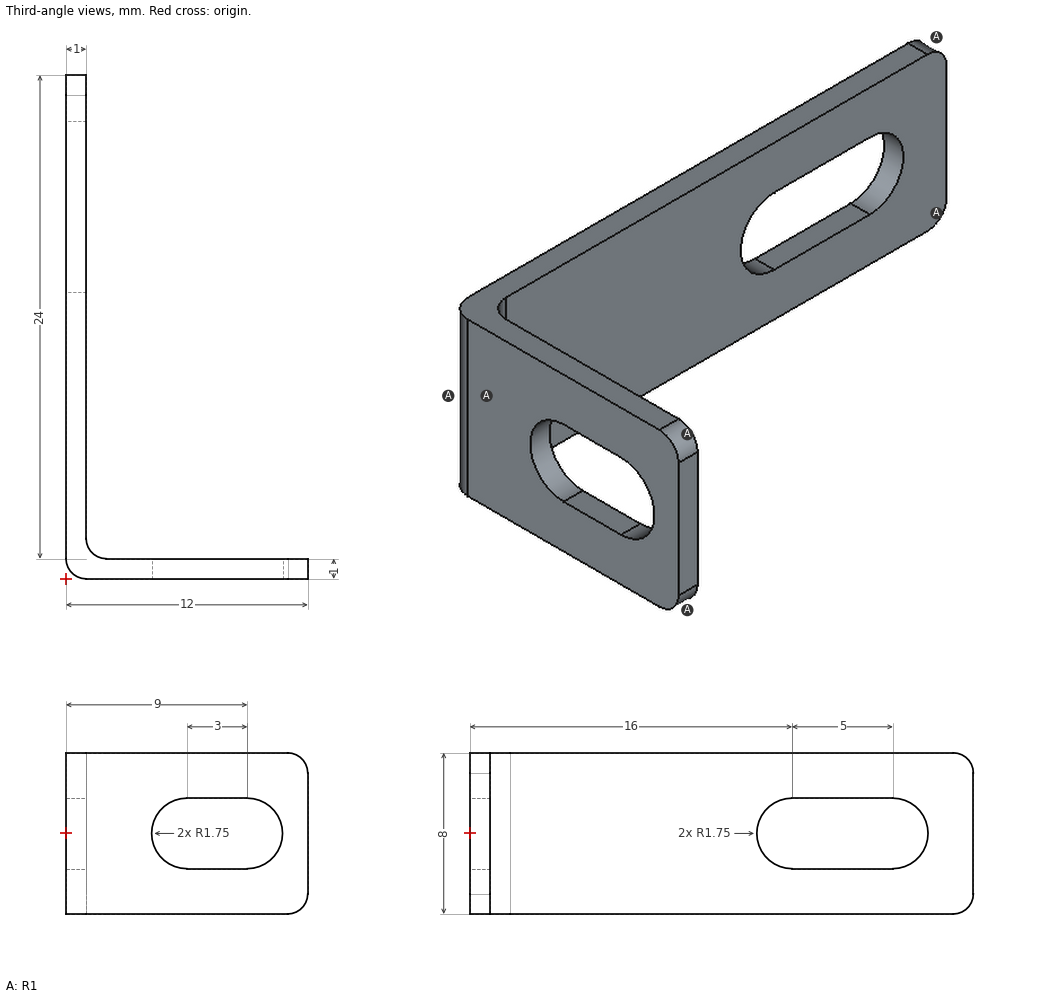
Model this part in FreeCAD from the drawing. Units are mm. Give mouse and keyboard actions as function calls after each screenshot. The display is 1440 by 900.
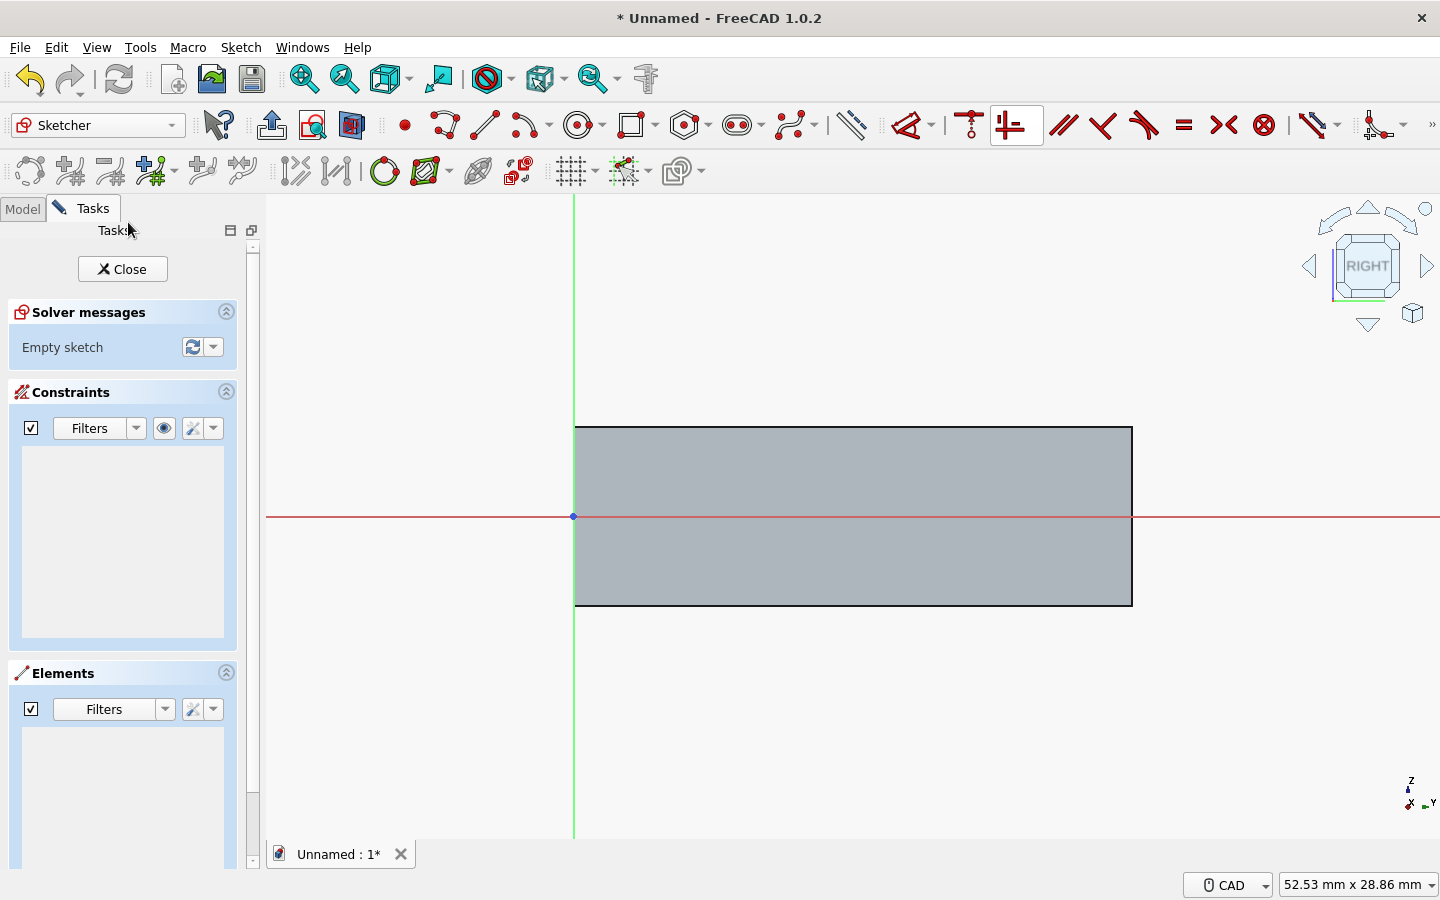
scroll(1074, 516, up, 6)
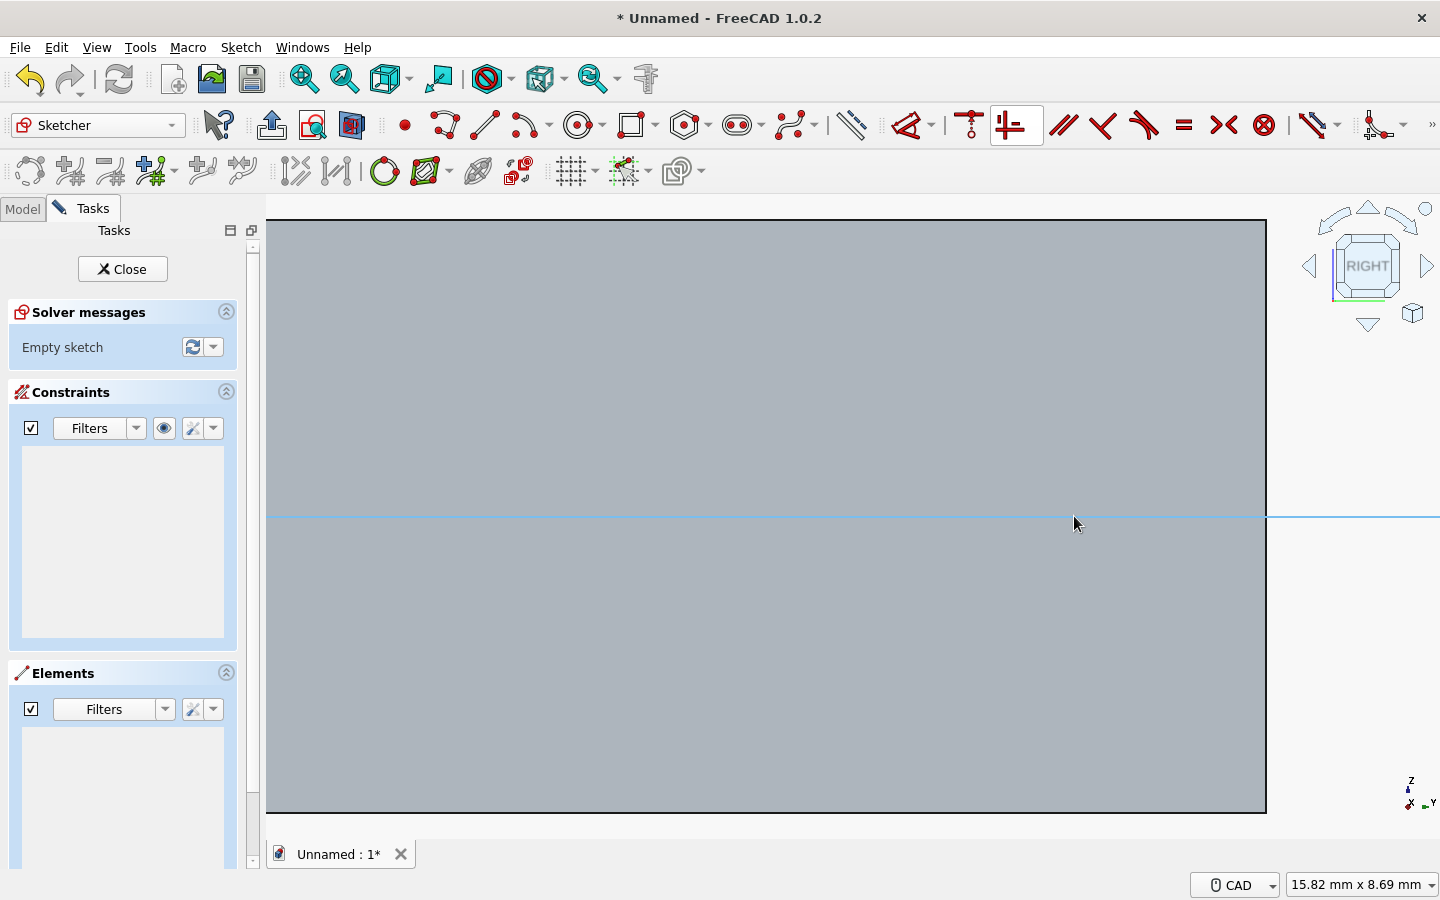
key(g)
key(s)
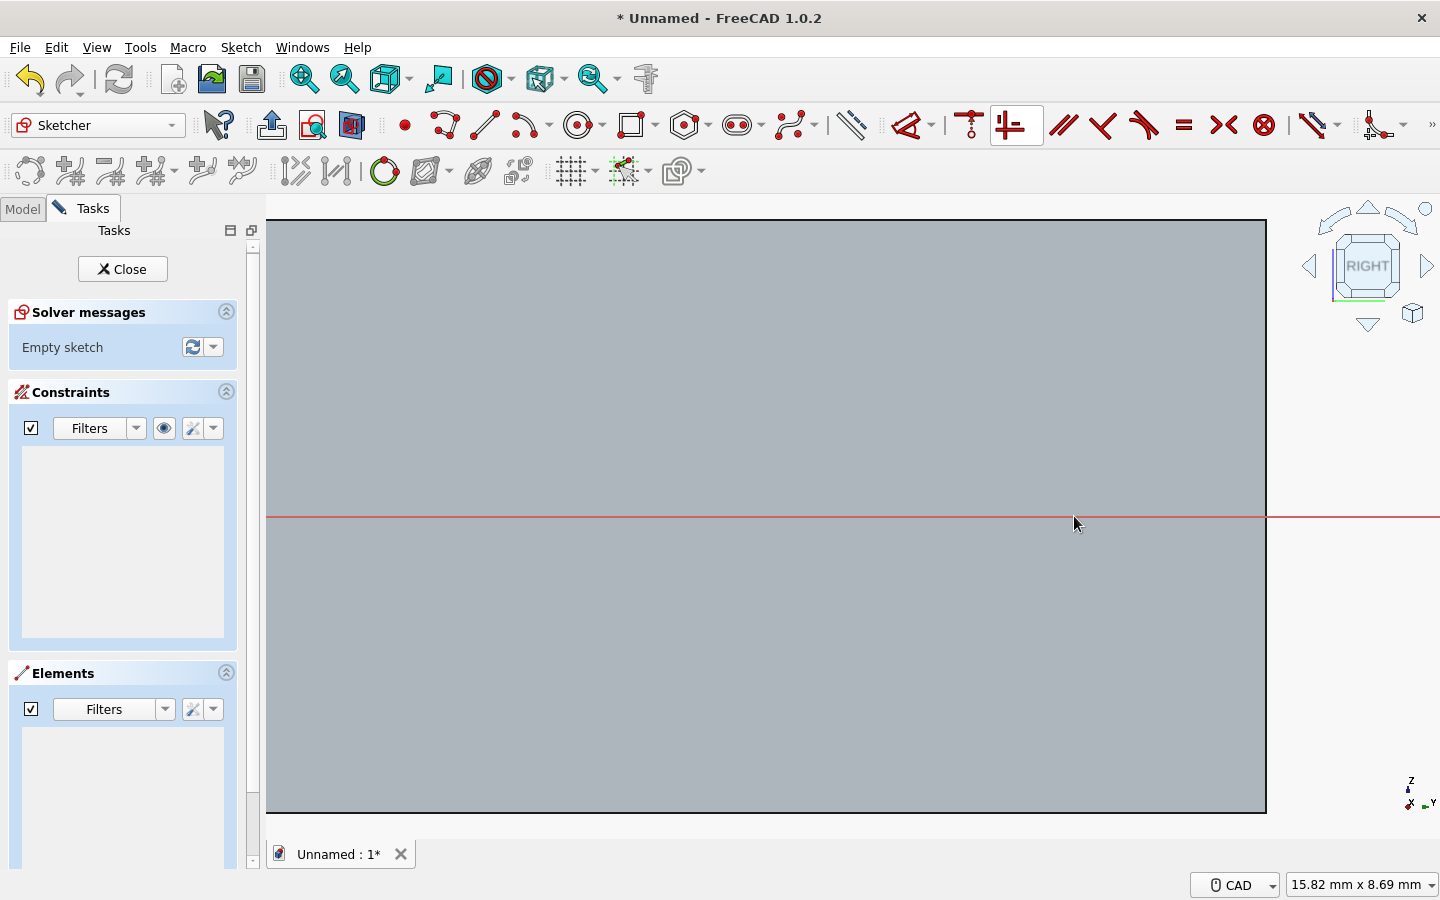
click(598, 516)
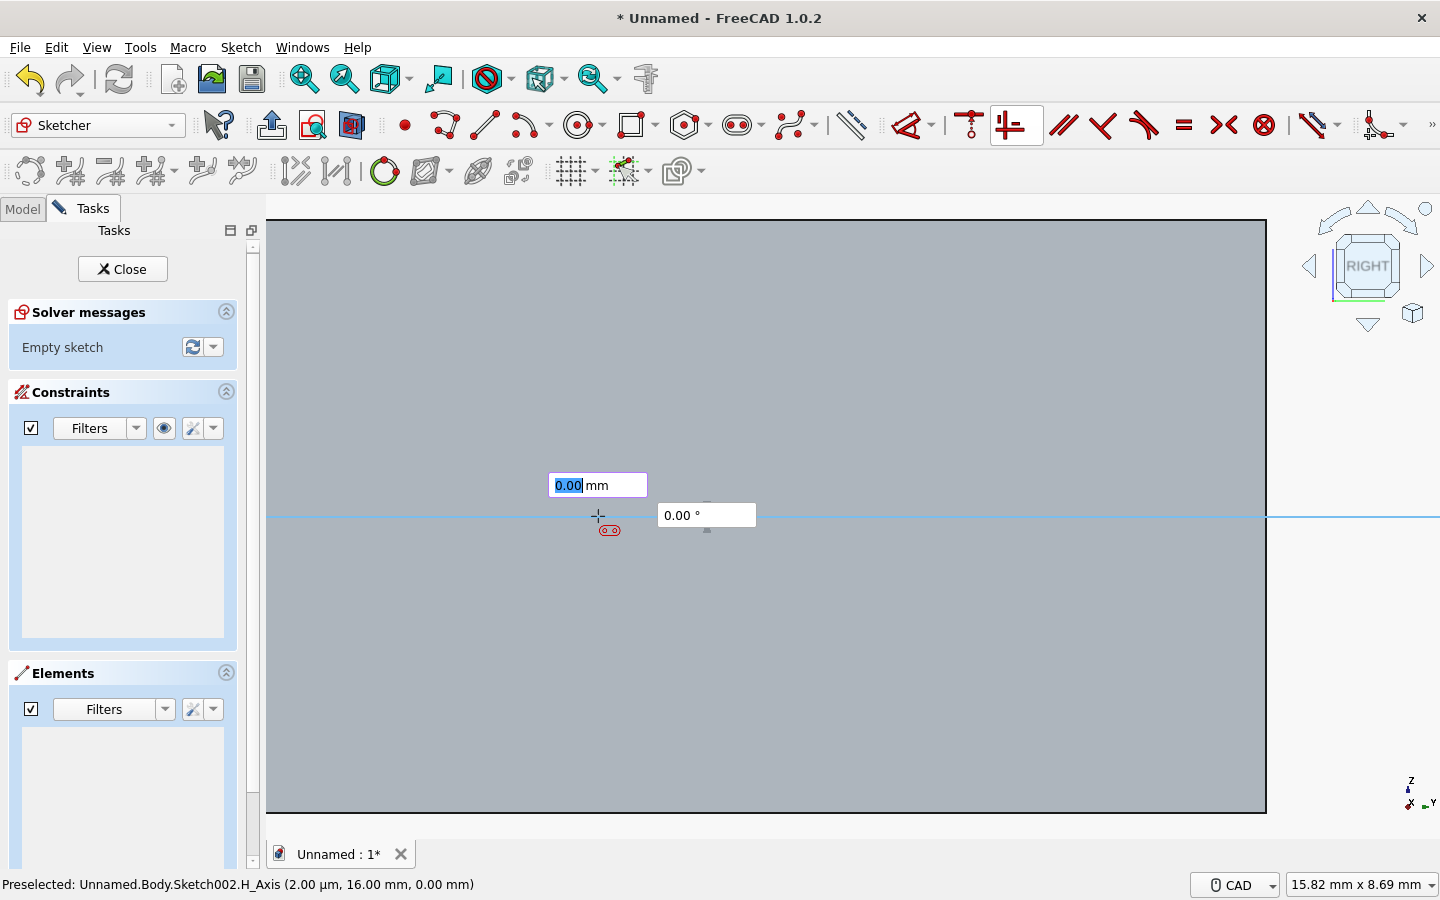
click(969, 508)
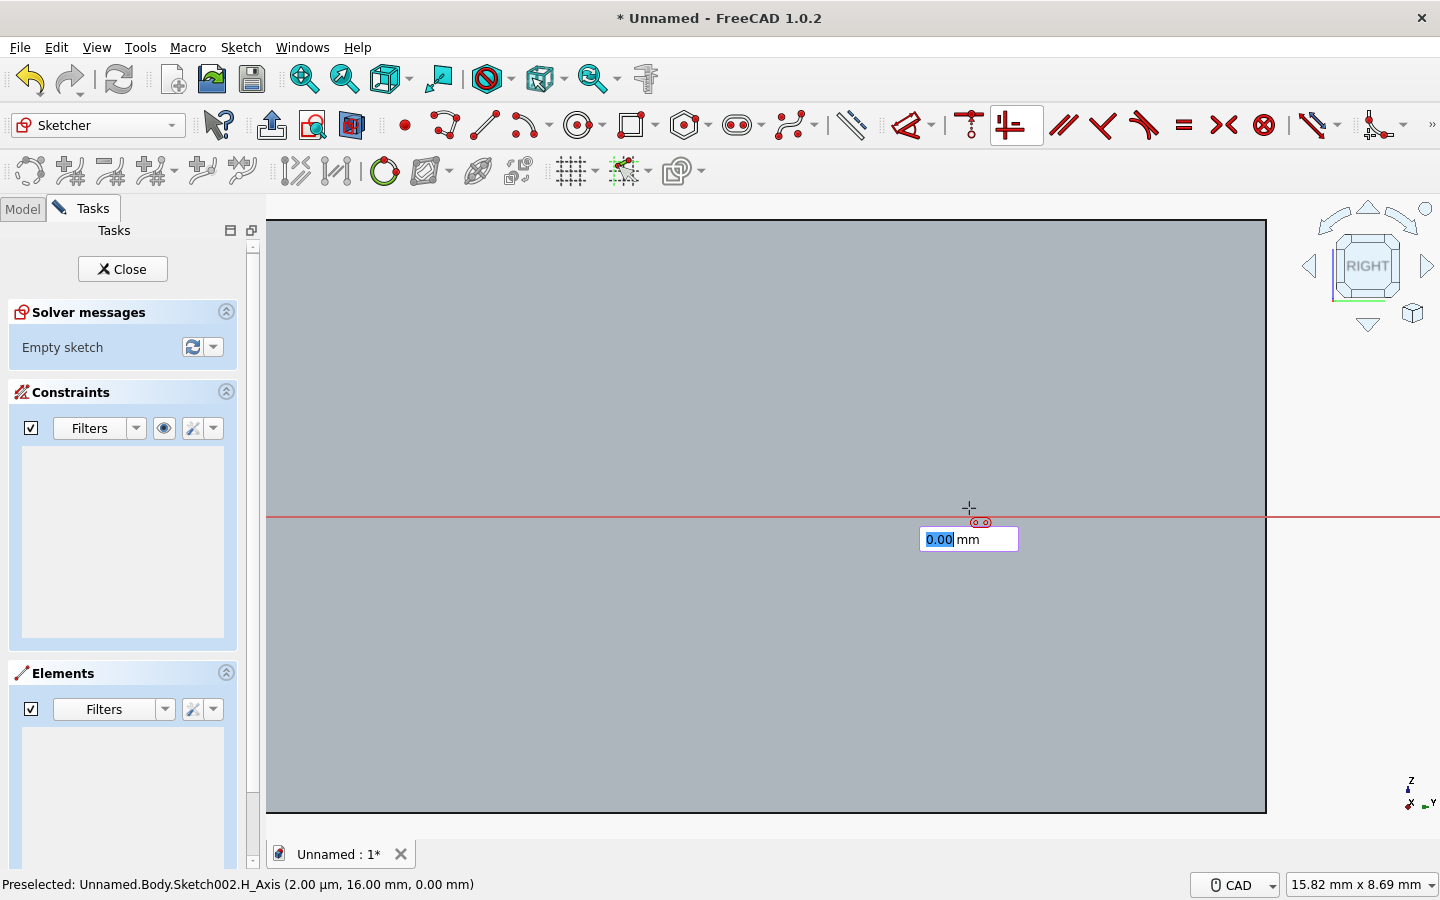
click(784, 646)
key(Escape)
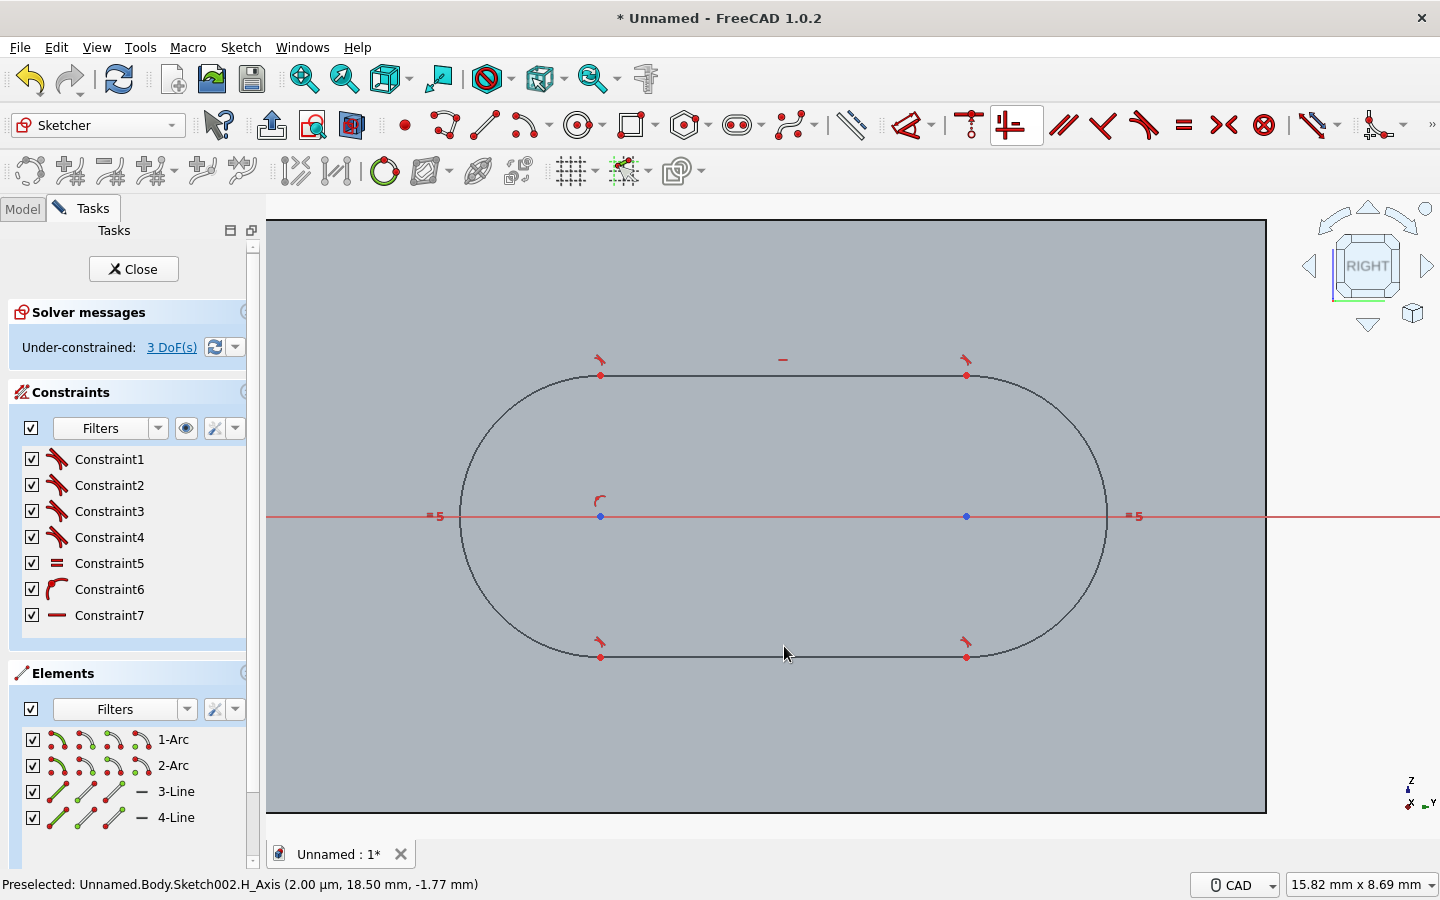
key(d)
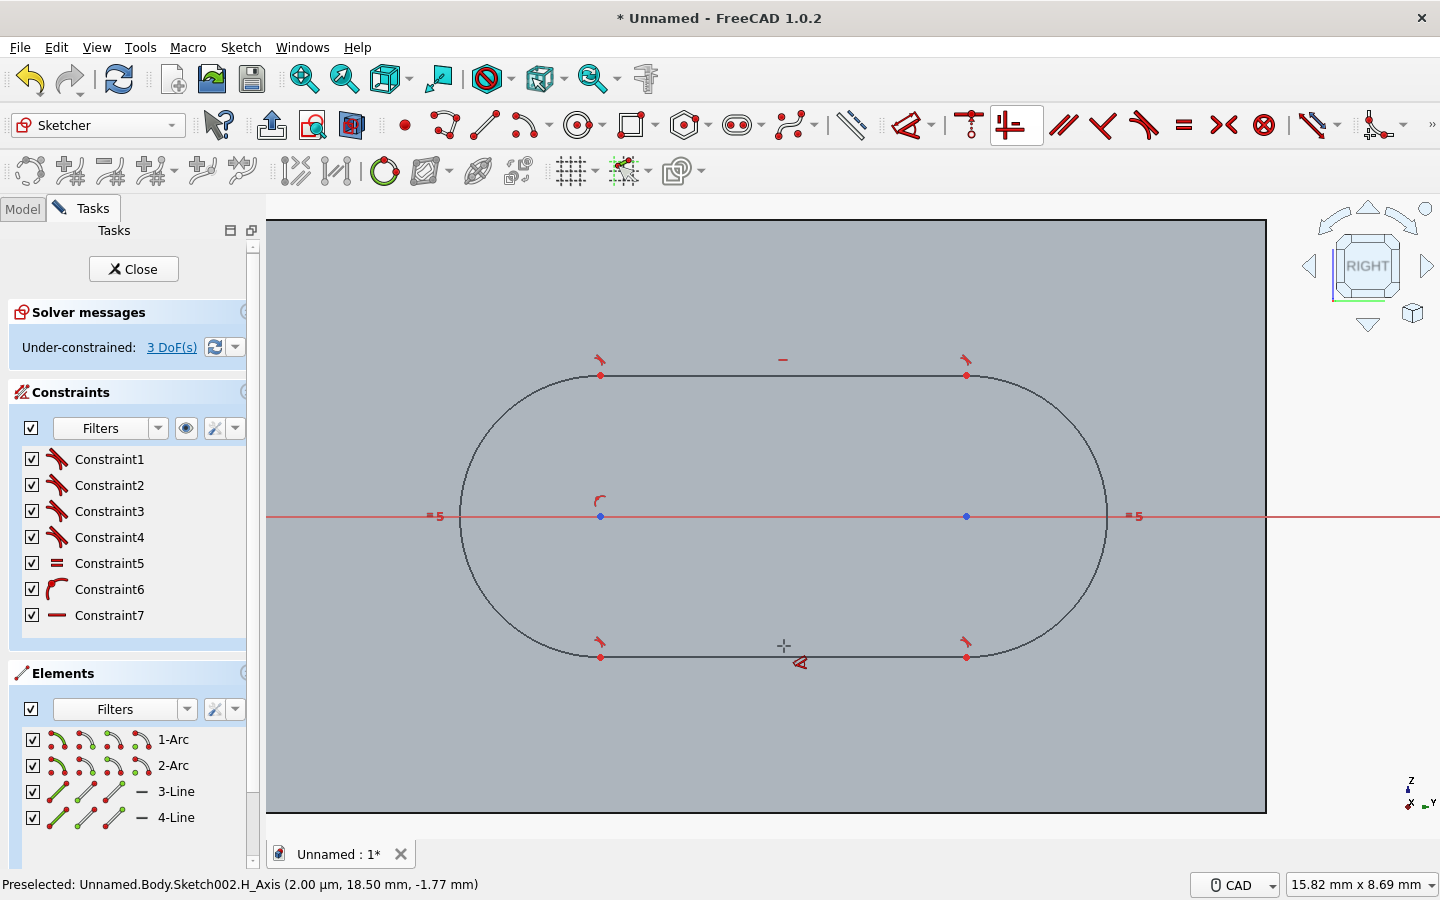
click(487, 434)
click(461, 415)